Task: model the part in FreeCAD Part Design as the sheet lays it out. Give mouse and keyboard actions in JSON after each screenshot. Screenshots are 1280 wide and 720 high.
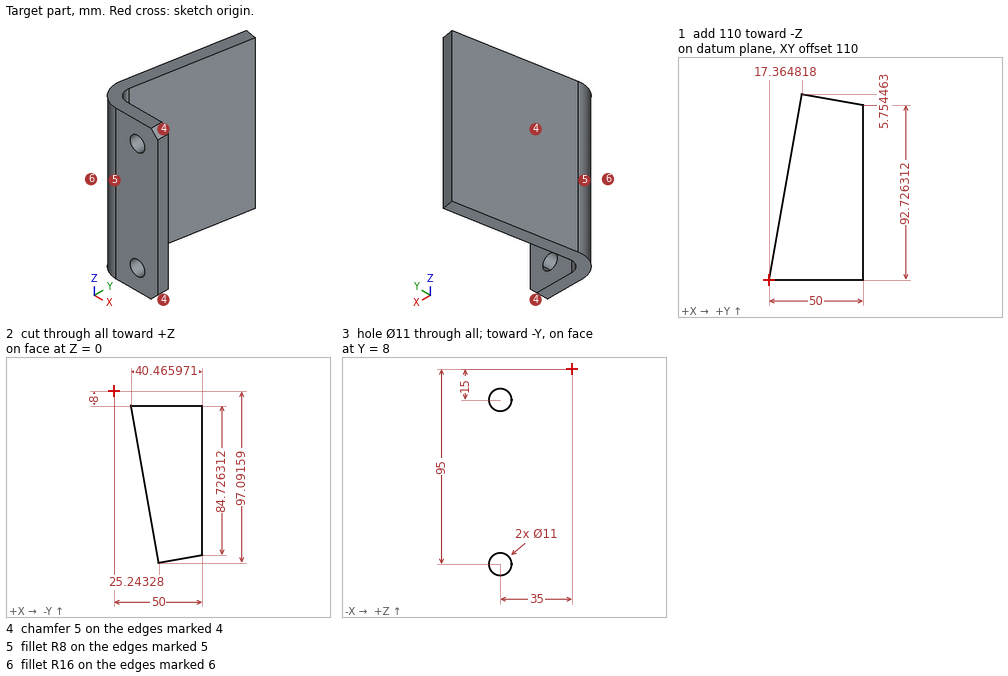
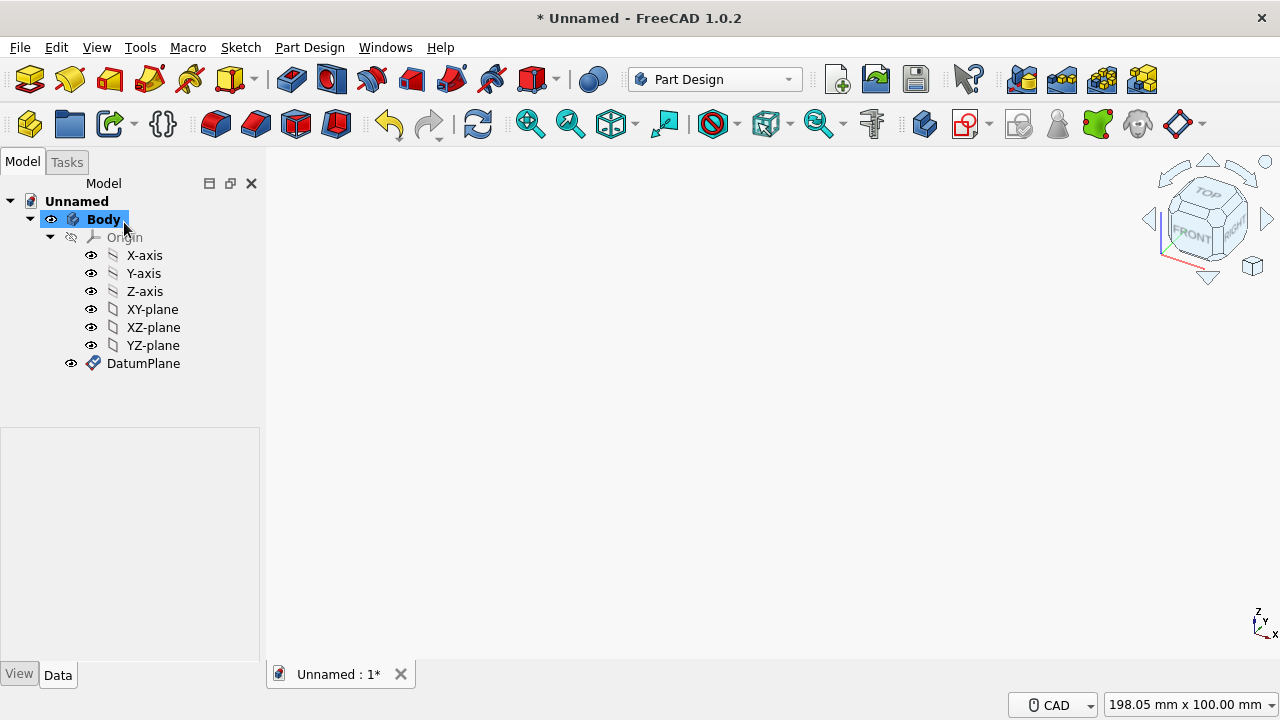
{"action": "left_click", "coordinate": [116, 363]}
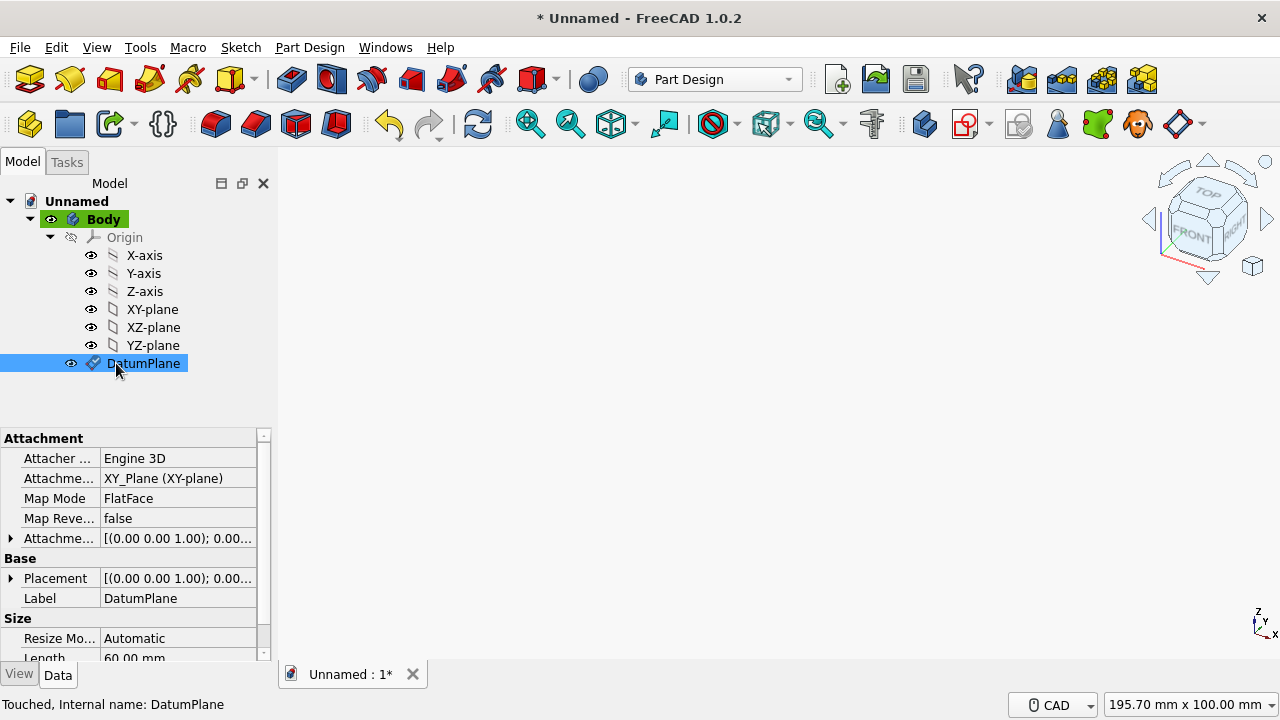
{"action": "left_click", "coordinate": [966, 124]}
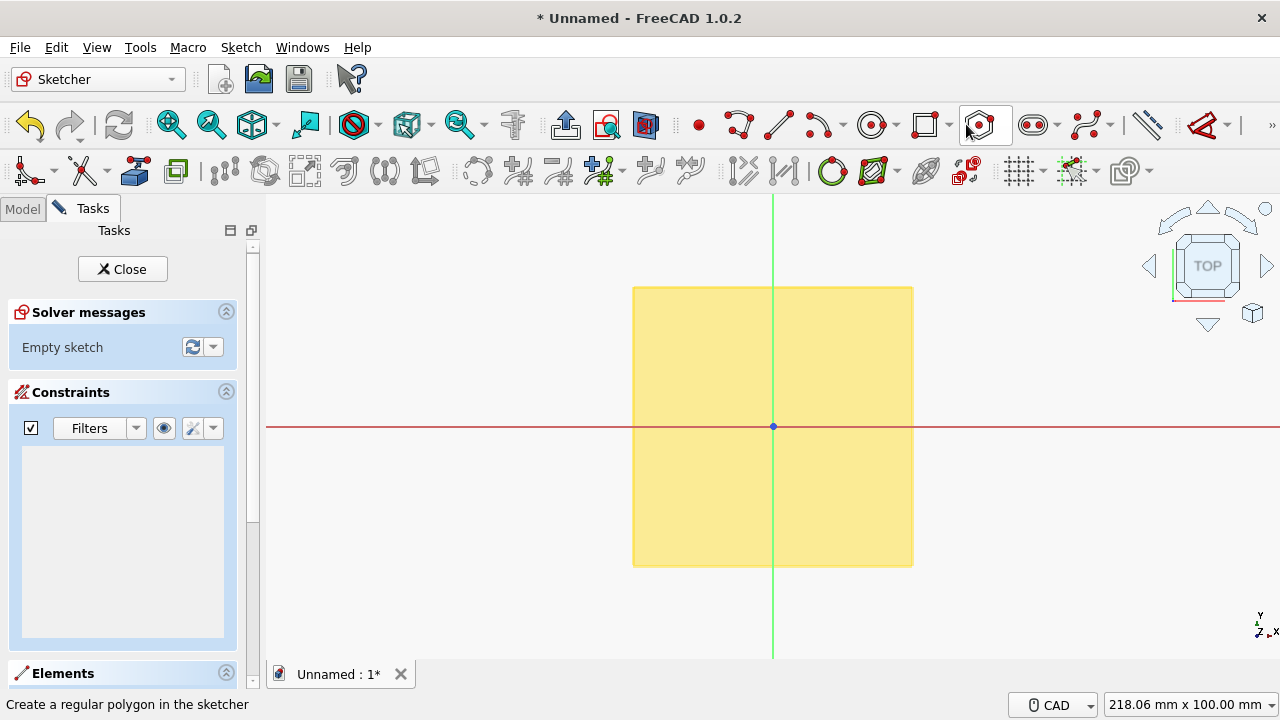
{"action": "scroll", "coordinate": [480, 631], "scroll_direction": "down", "scroll_amount": 3}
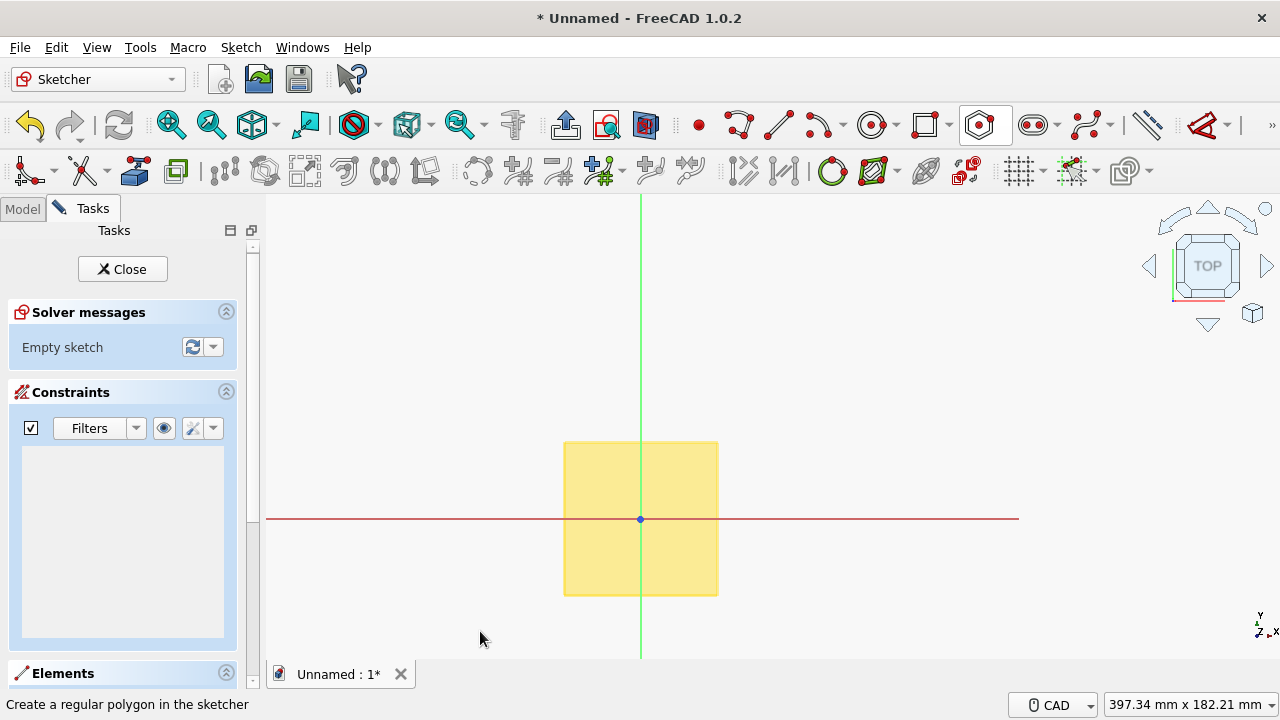
{"action": "left_click", "coordinate": [740, 126]}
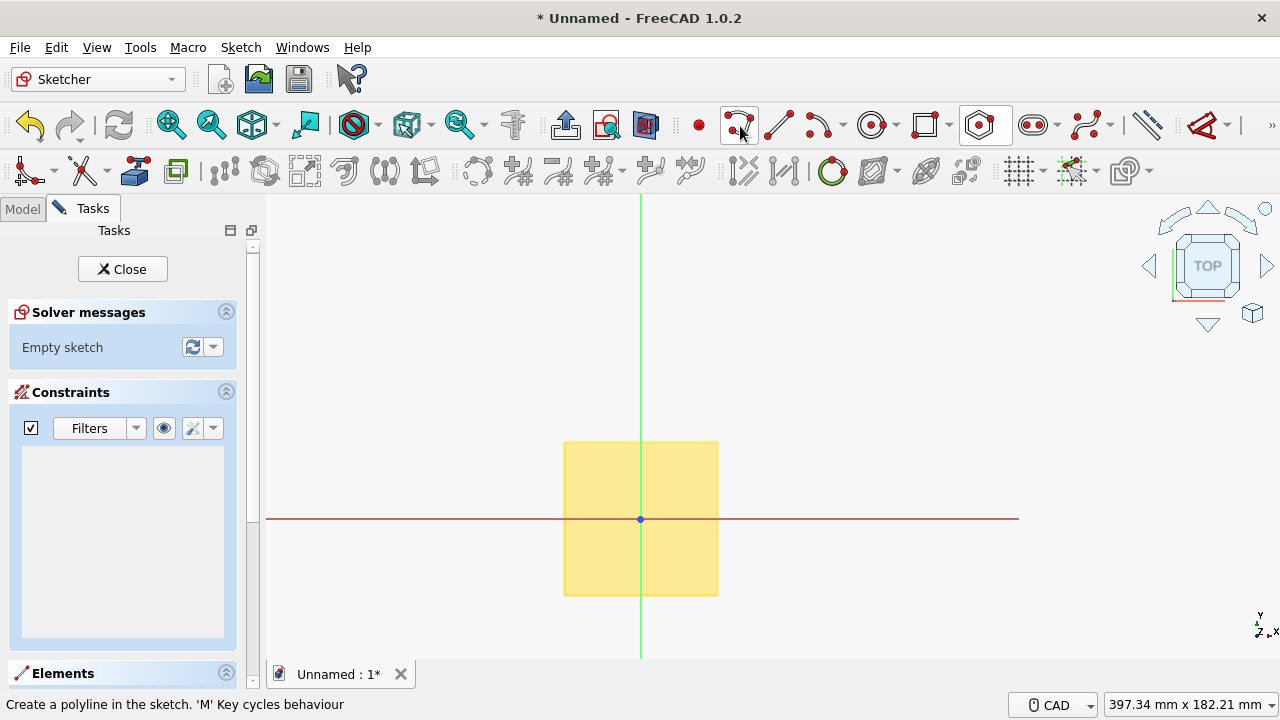
{"action": "left_click", "coordinate": [641, 519]}
{"action": "left_click", "coordinate": [768, 510]}
{"action": "left_click", "coordinate": [768, 283]}
{"action": "left_click", "coordinate": [685, 268]}
{"action": "left_click", "coordinate": [641, 519]}
{"action": "key", "text": "Escape"}
{"action": "key", "text": "Escape"}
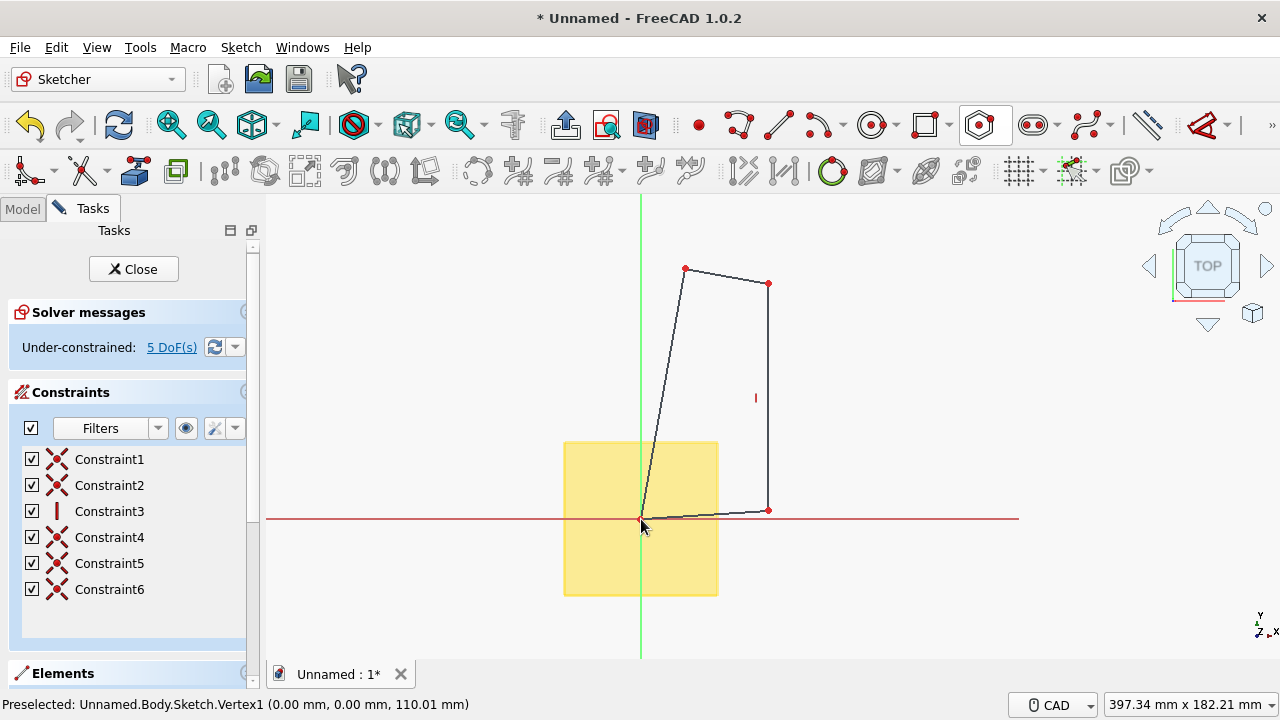
{"action": "left_click", "coordinate": [679, 517]}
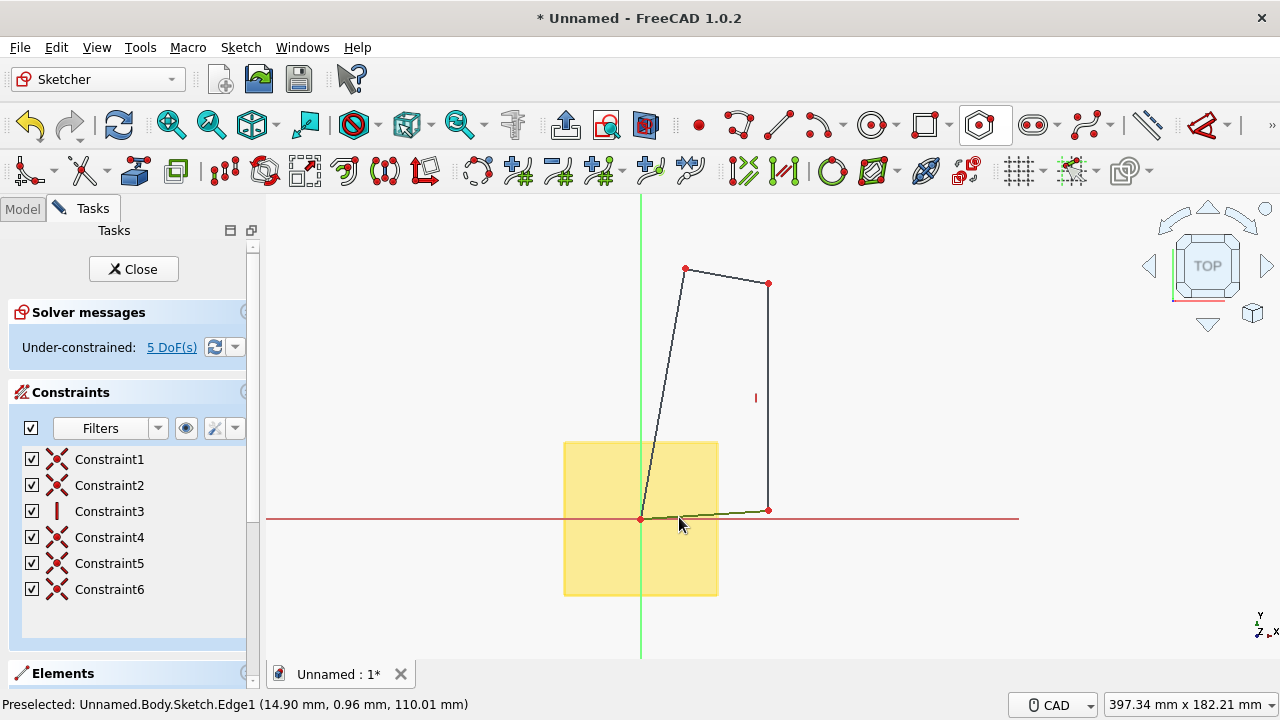
{"action": "key", "text": "h"}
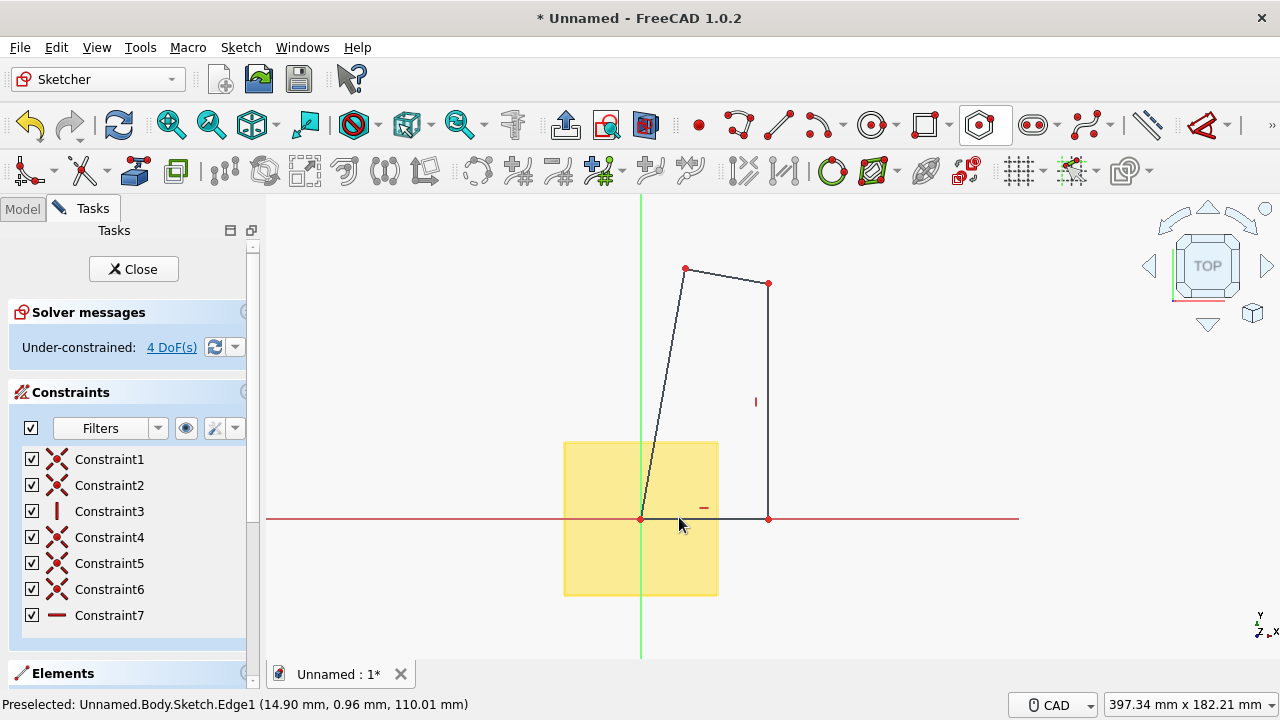
{"action": "left_click", "coordinate": [1202, 126]}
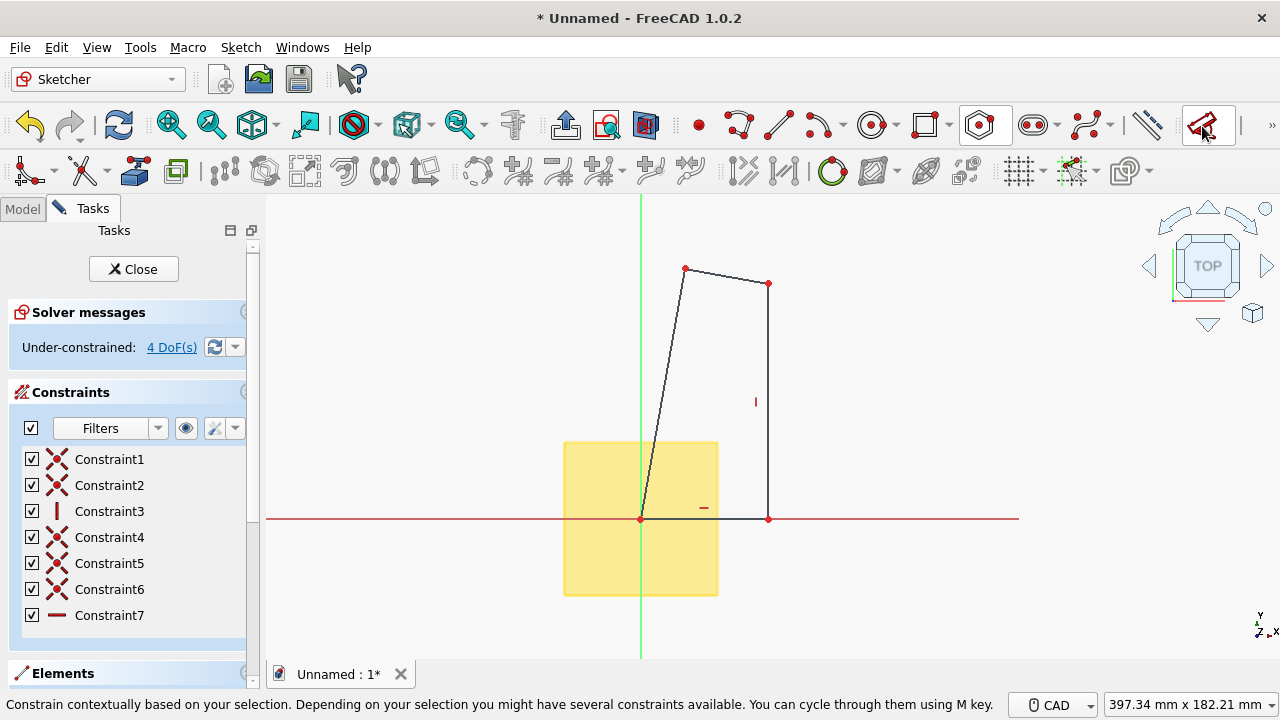
{"action": "left_click", "coordinate": [679, 519]}
{"action": "left_click", "coordinate": [704, 553]}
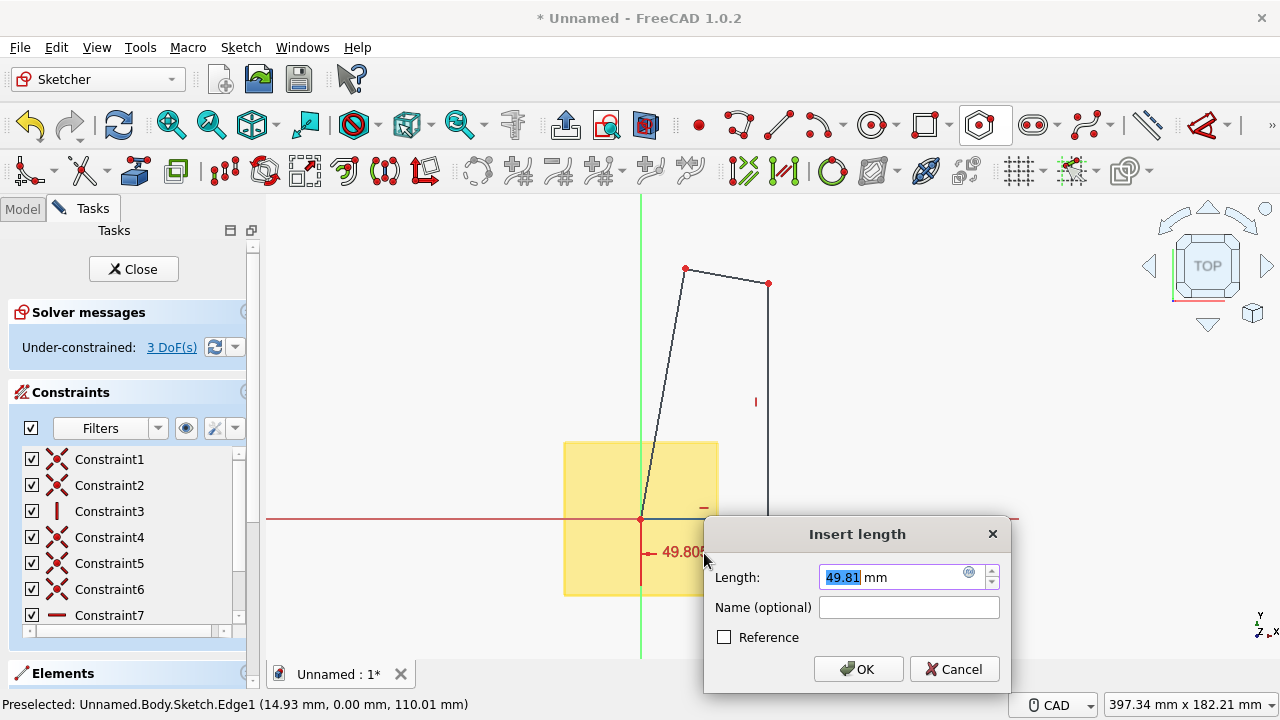
{"action": "type", "text": "50"}
{"action": "key", "text": "Return"}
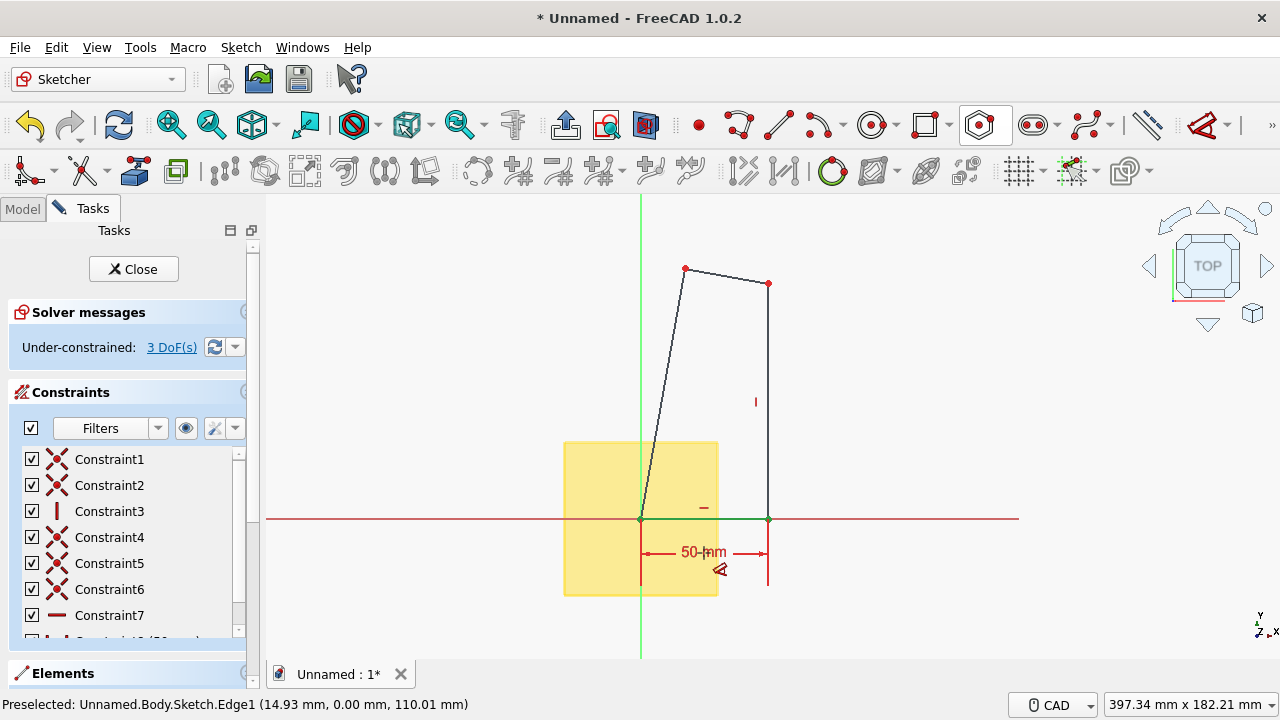
{"action": "left_click", "coordinate": [768, 449]}
{"action": "left_click", "coordinate": [802, 402]}